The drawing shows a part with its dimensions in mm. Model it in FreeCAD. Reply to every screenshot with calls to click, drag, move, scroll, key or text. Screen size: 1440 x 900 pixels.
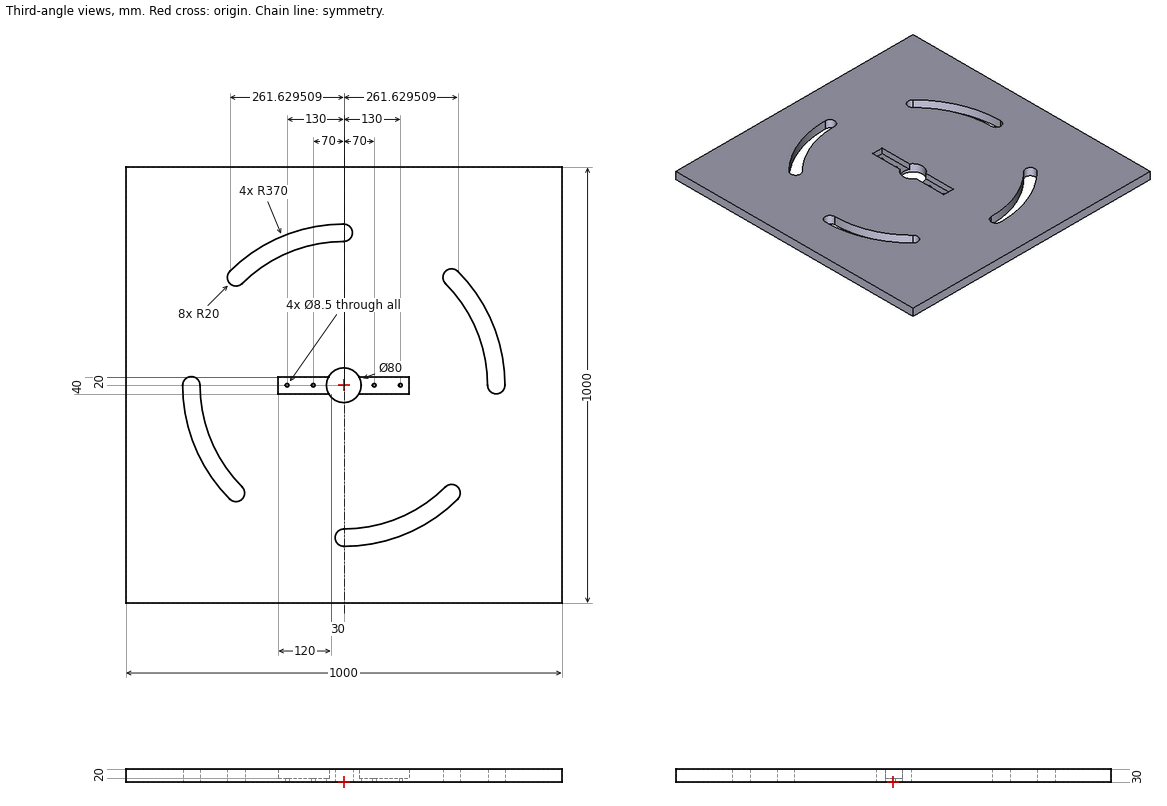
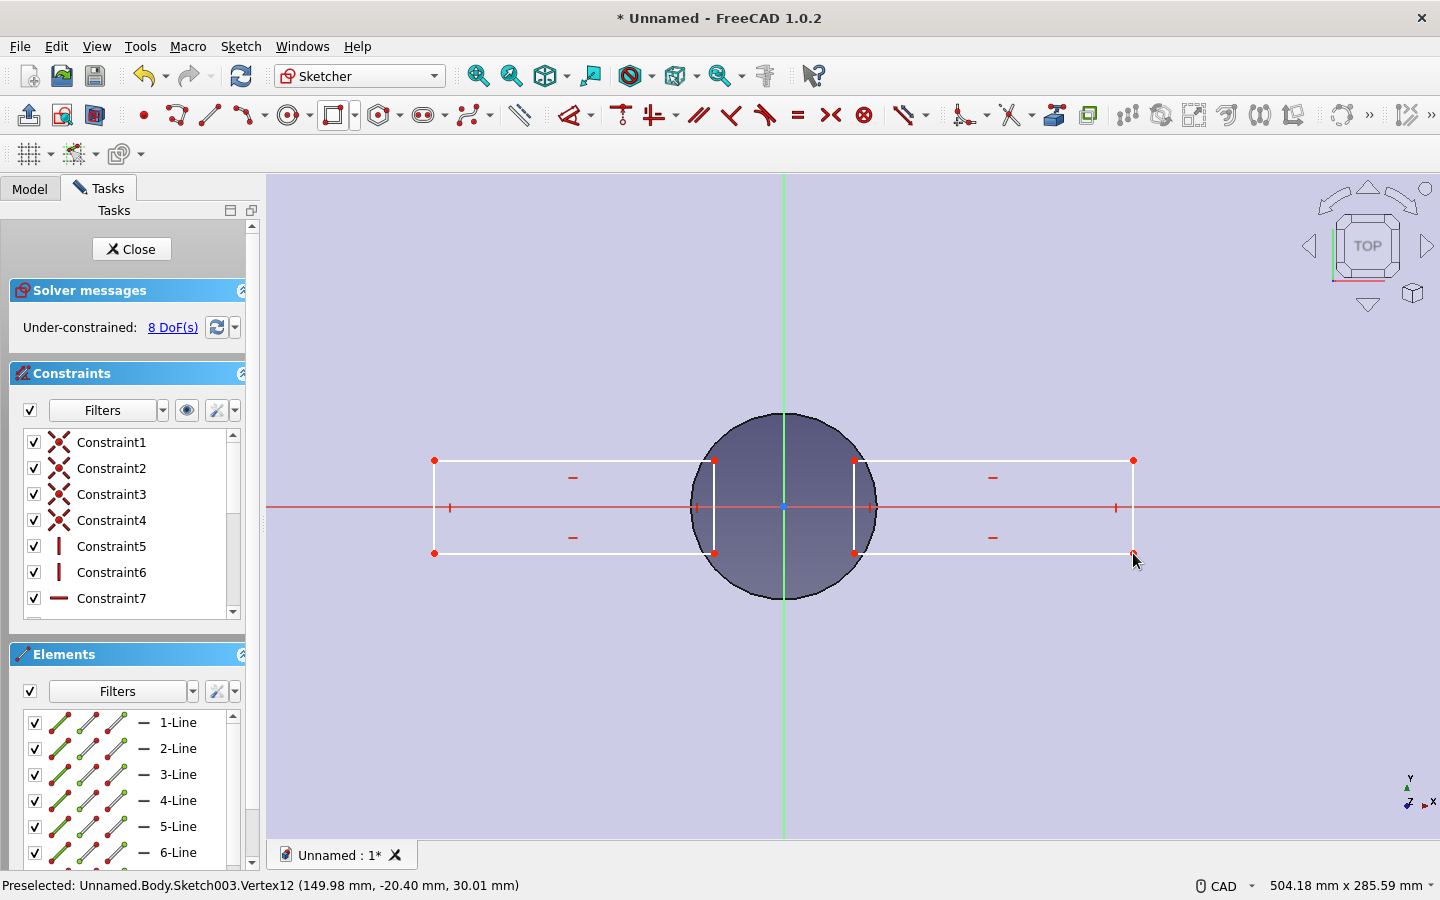
click(714, 461)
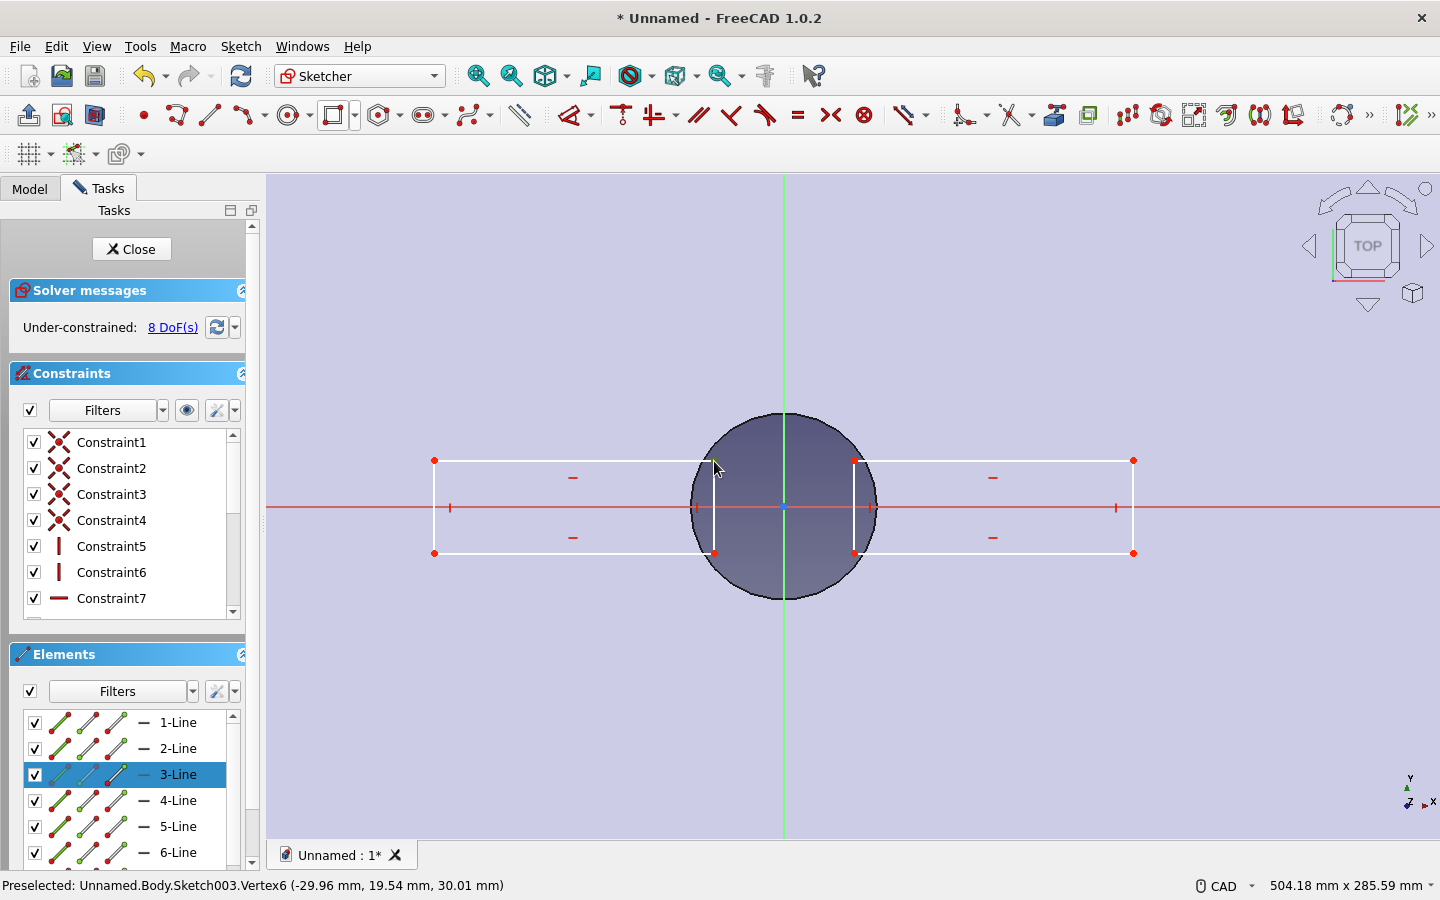
click(854, 461)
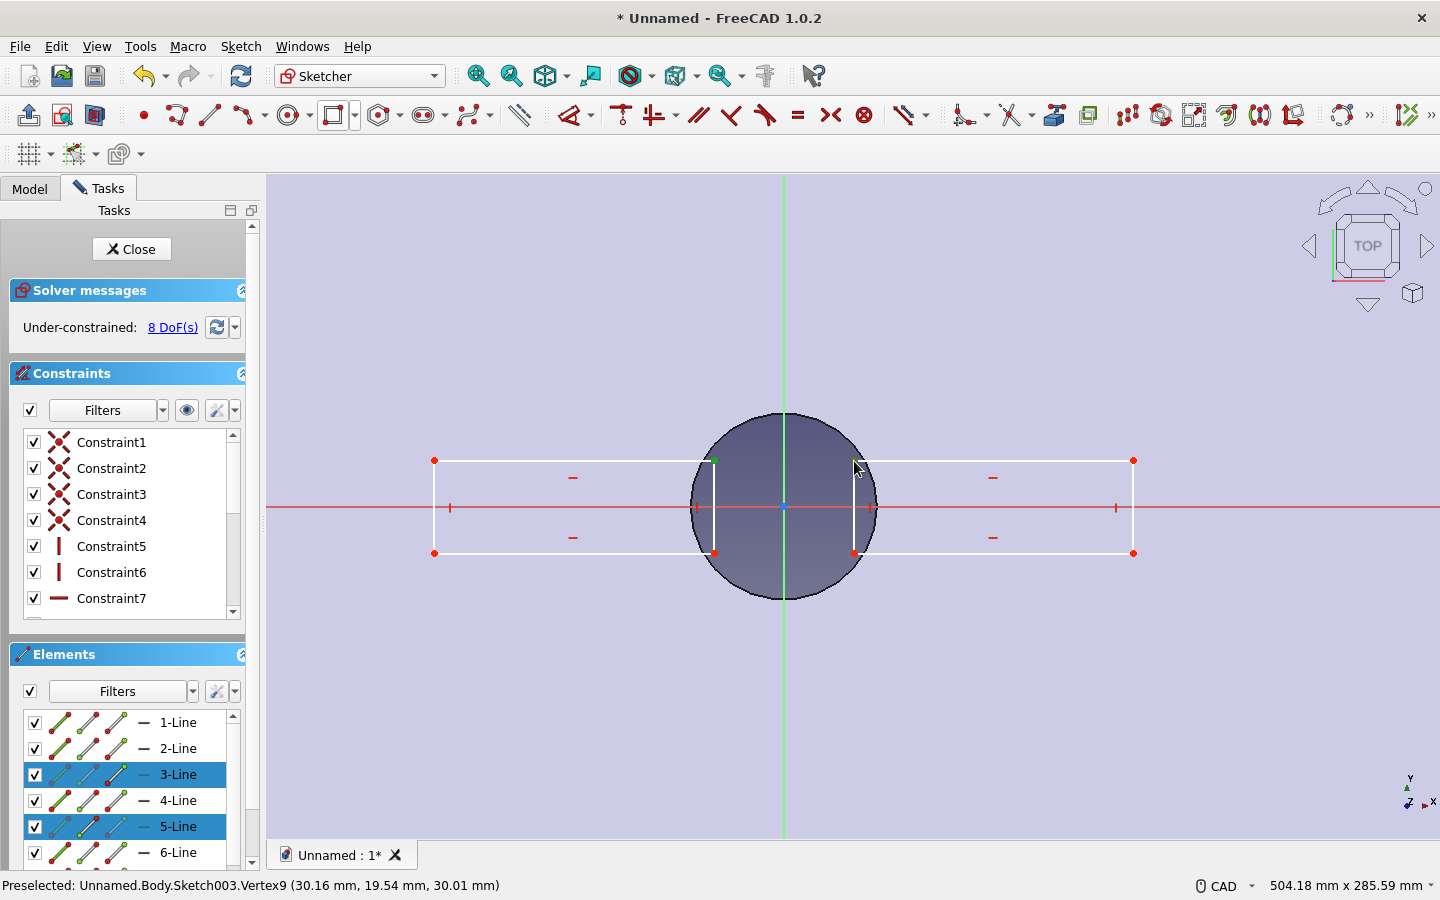
click(784, 768)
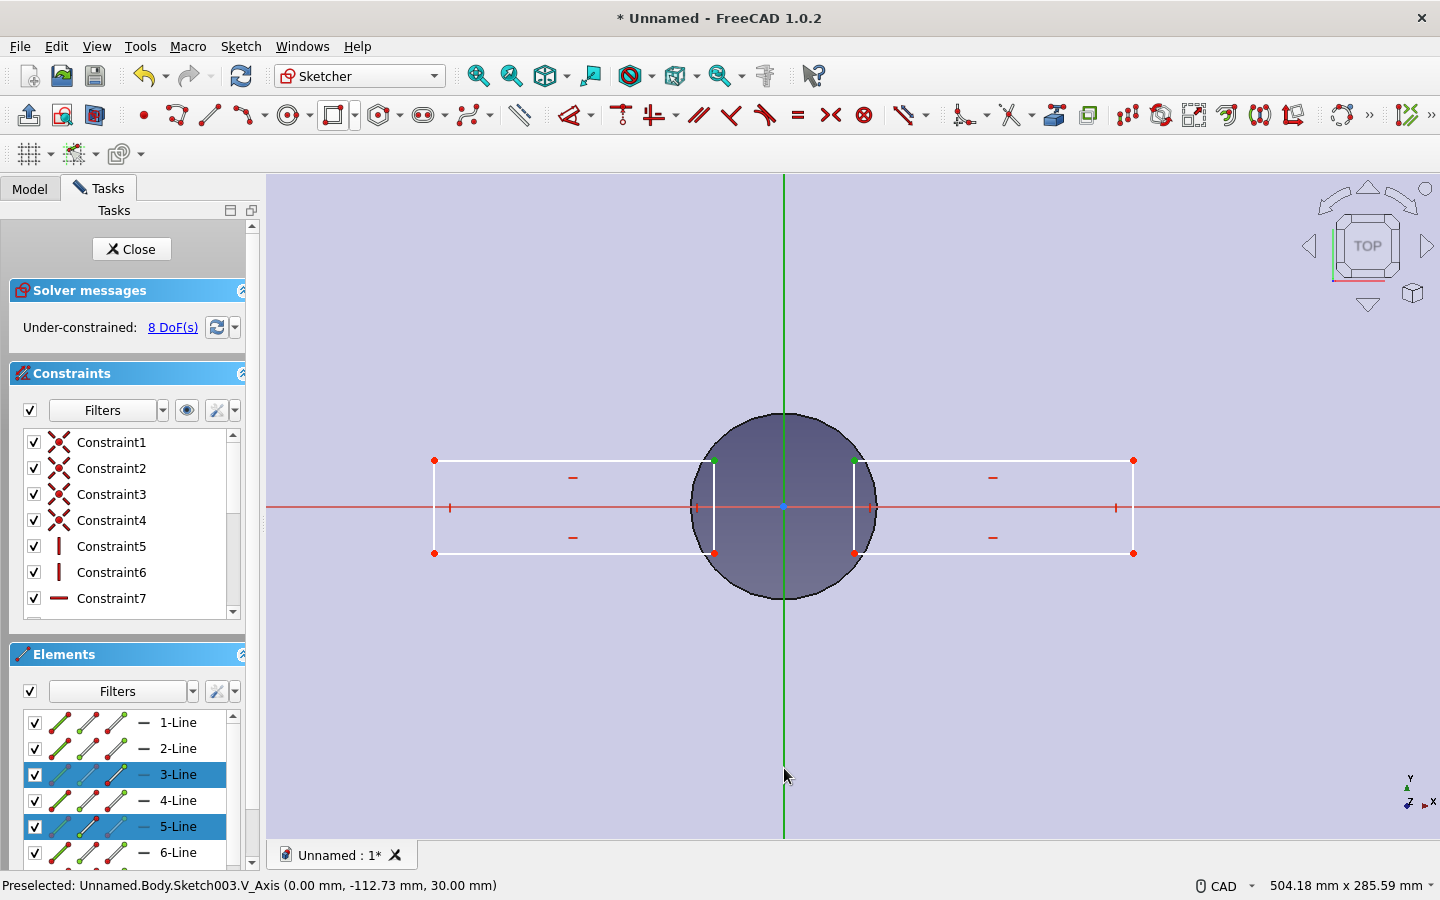
click(831, 116)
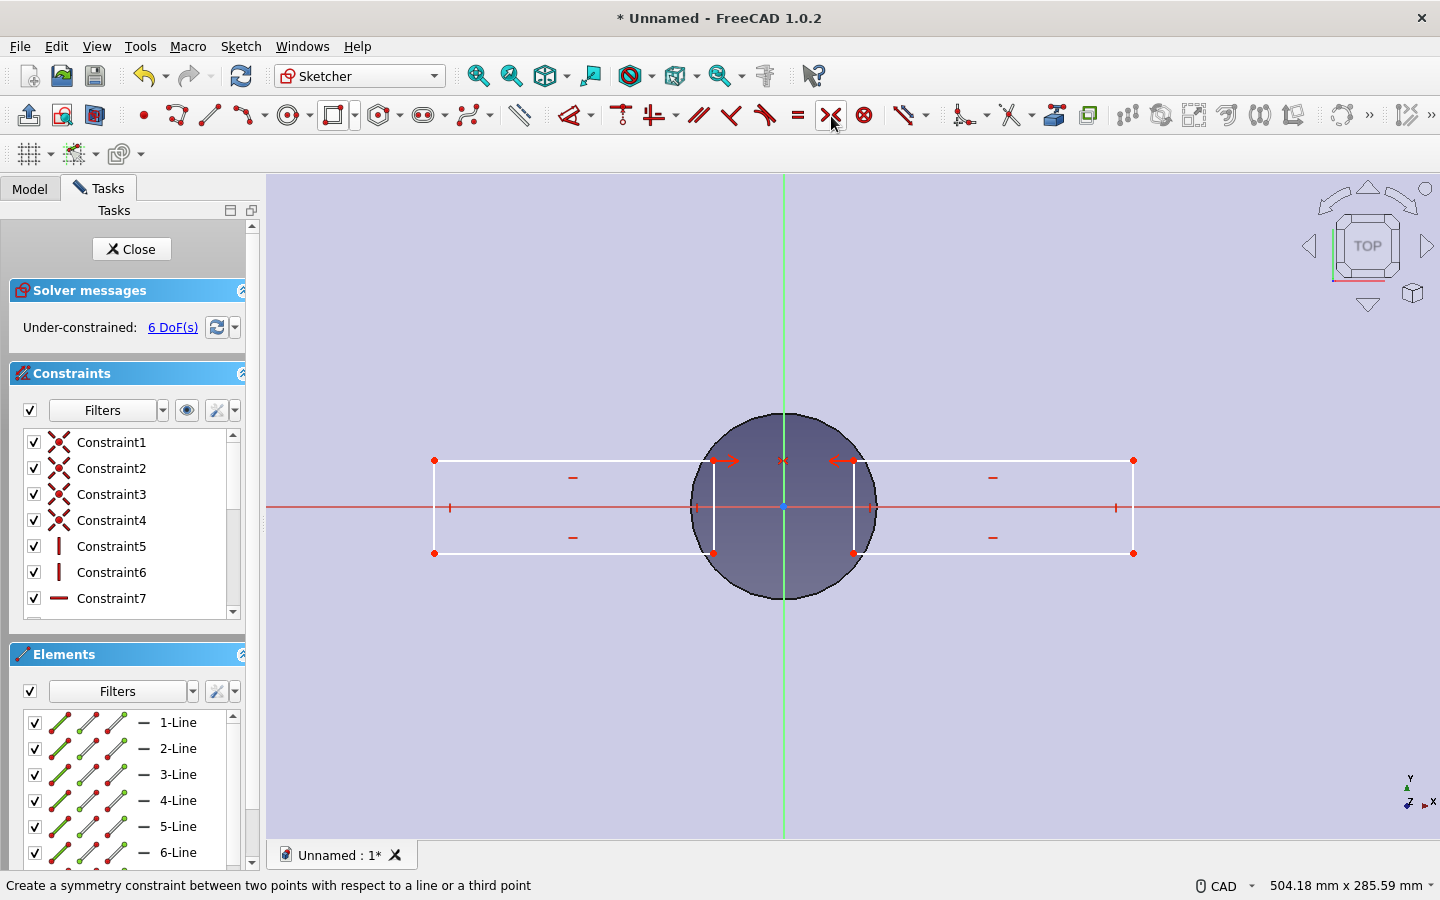
click(434, 554)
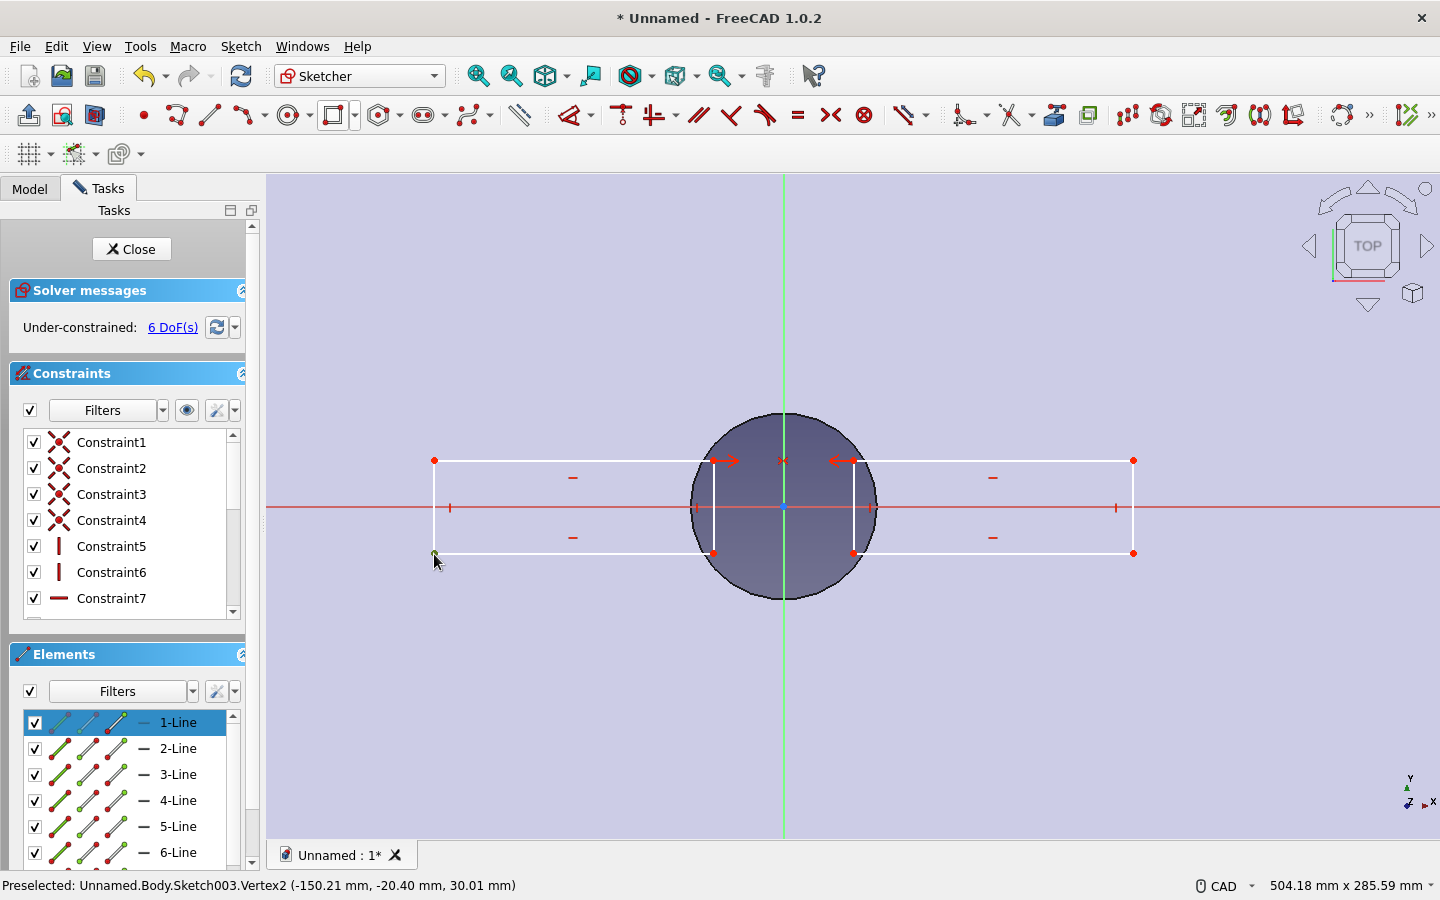
click(1133, 554)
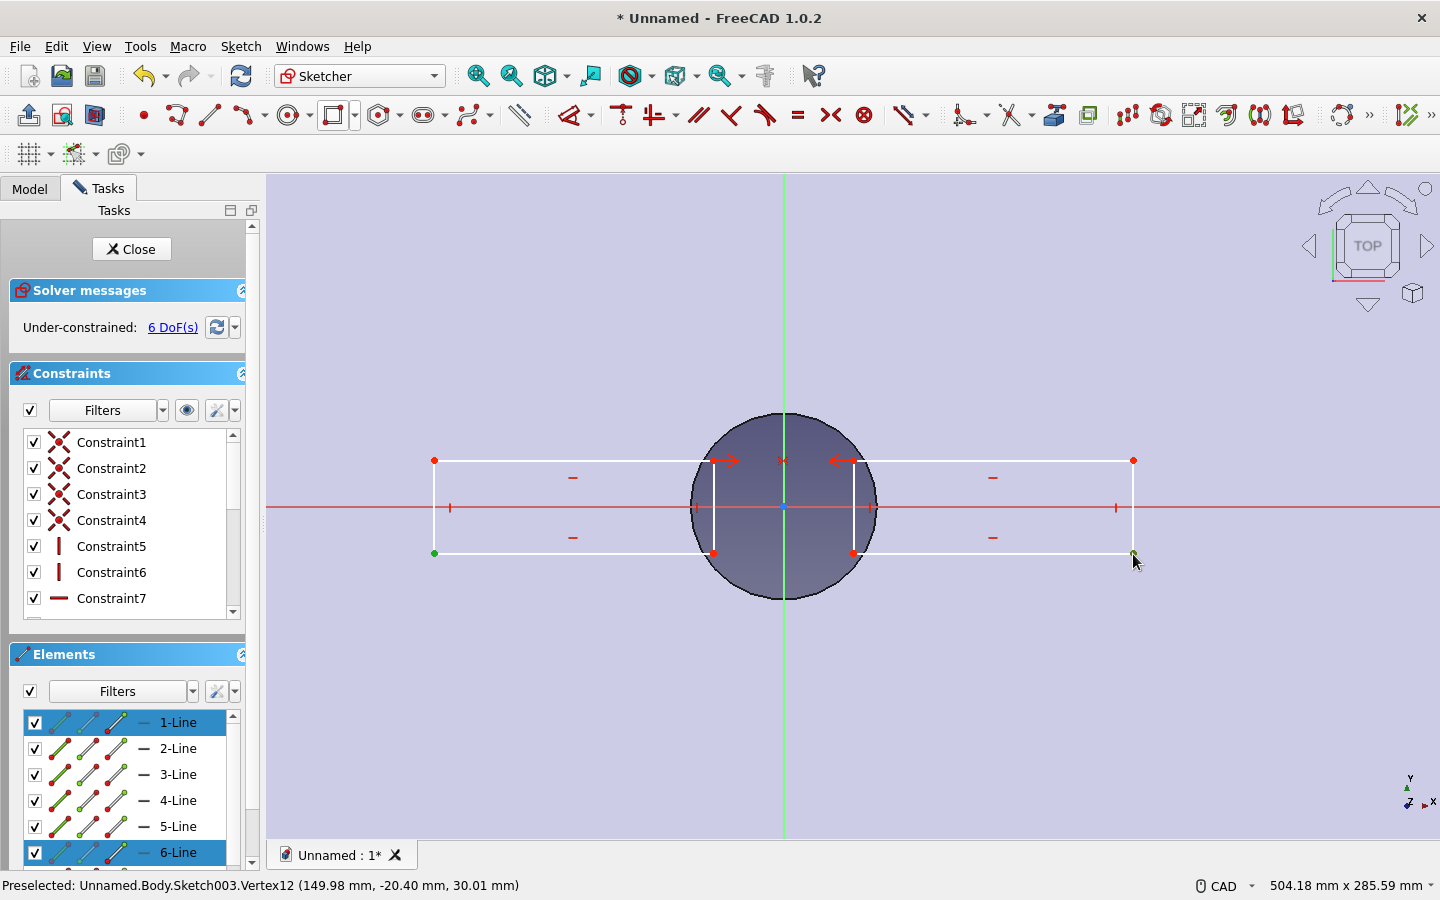
click(784, 768)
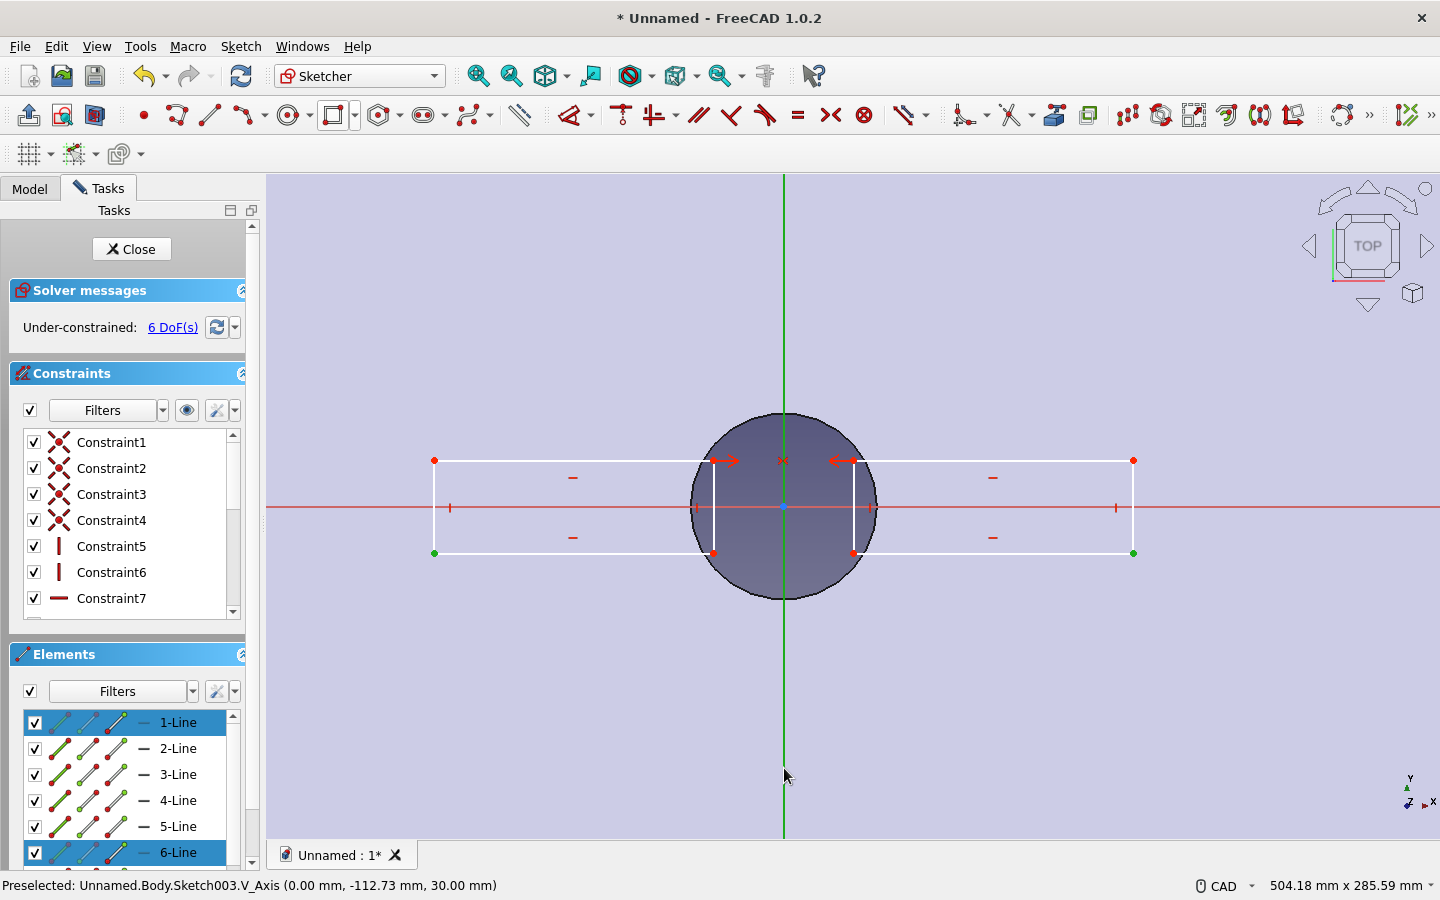
key(s)